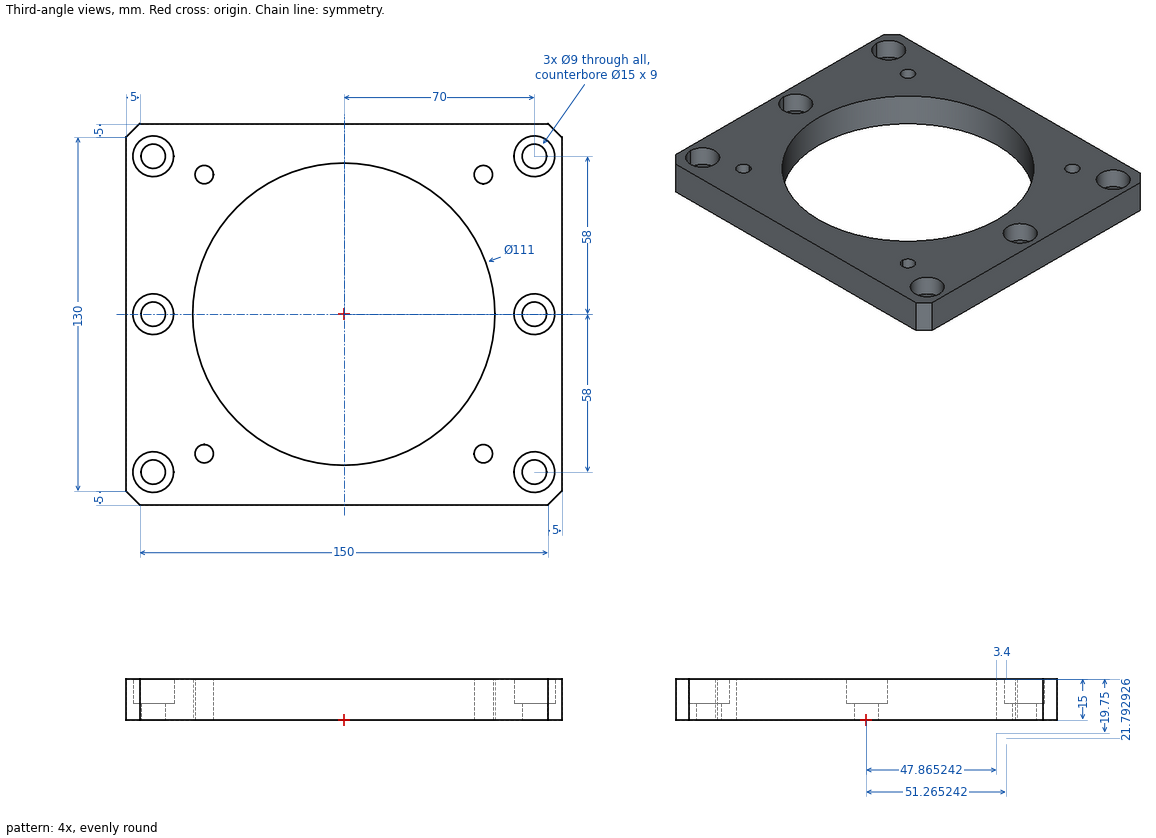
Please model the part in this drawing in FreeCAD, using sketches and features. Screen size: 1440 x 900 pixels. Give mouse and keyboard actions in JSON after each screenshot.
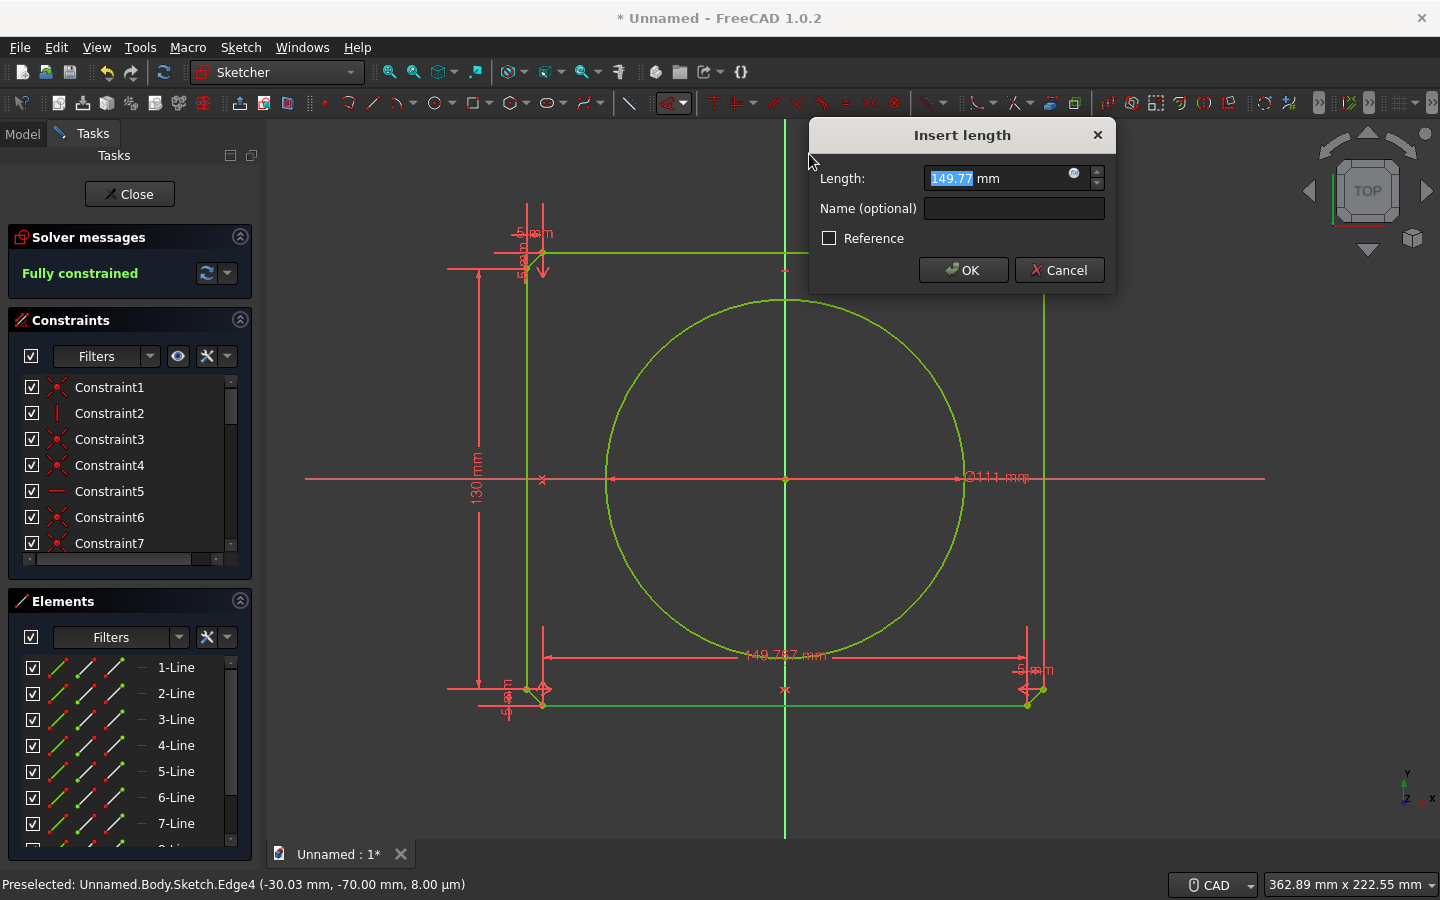
{"action": "type", "text": "150"}
{"action": "key", "text": "Return"}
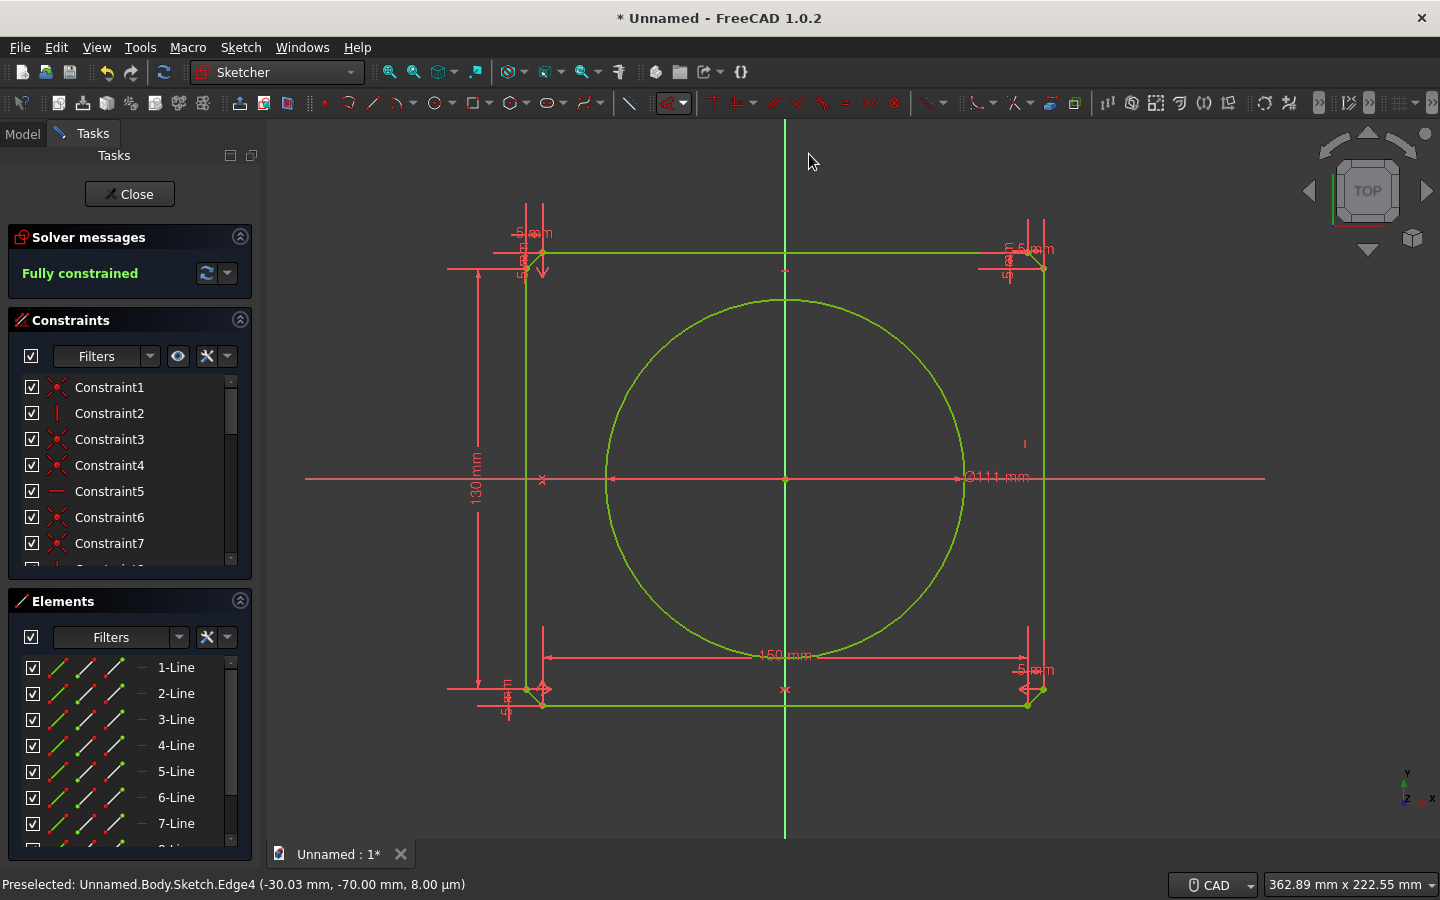
{"action": "left_click", "coordinate": [130, 194]}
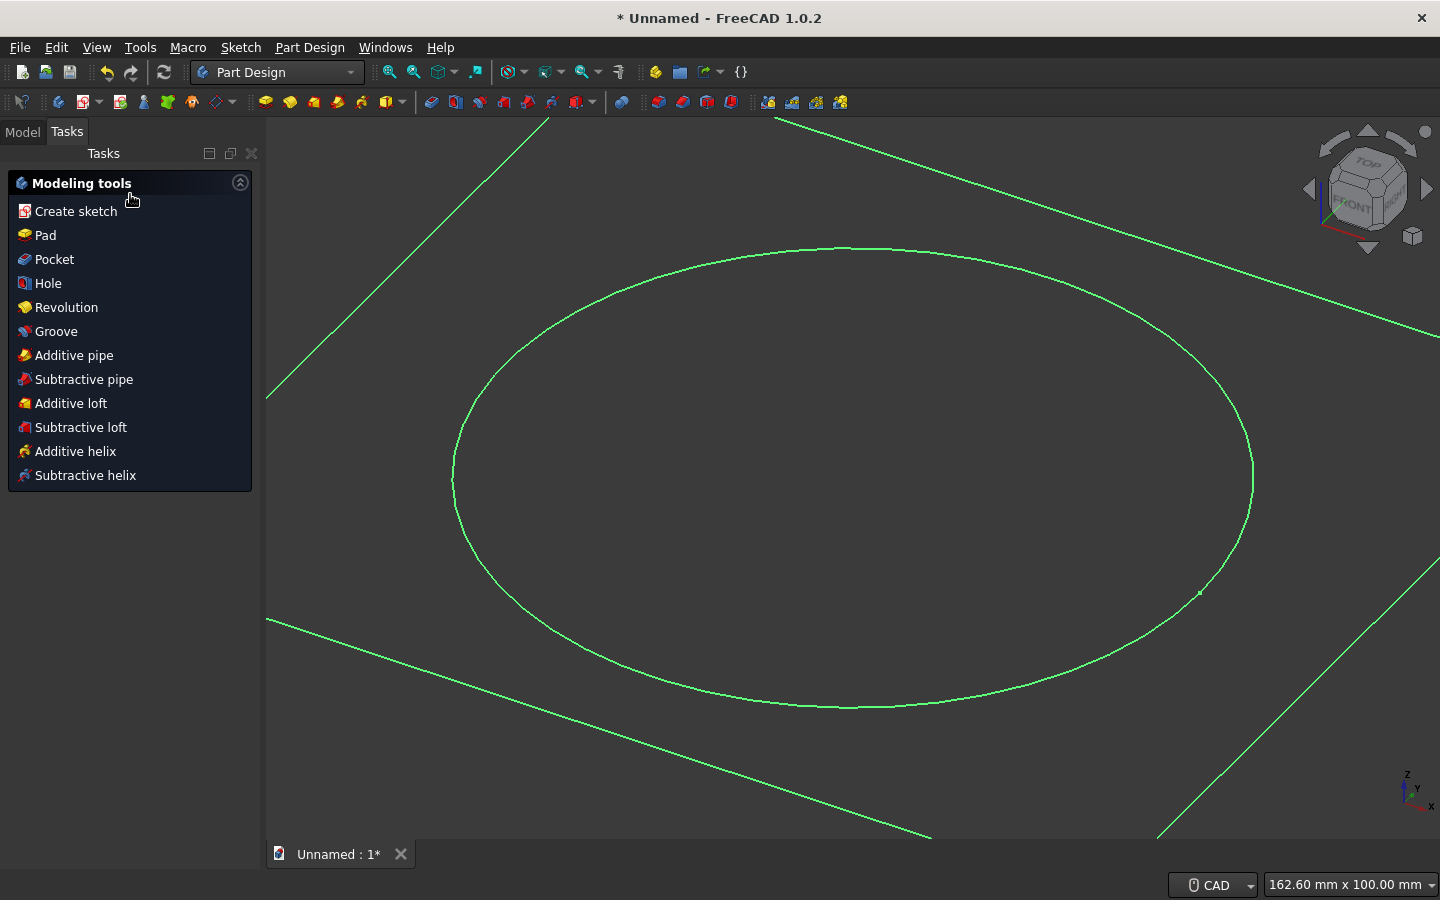
{"action": "left_click", "coordinate": [266, 102]}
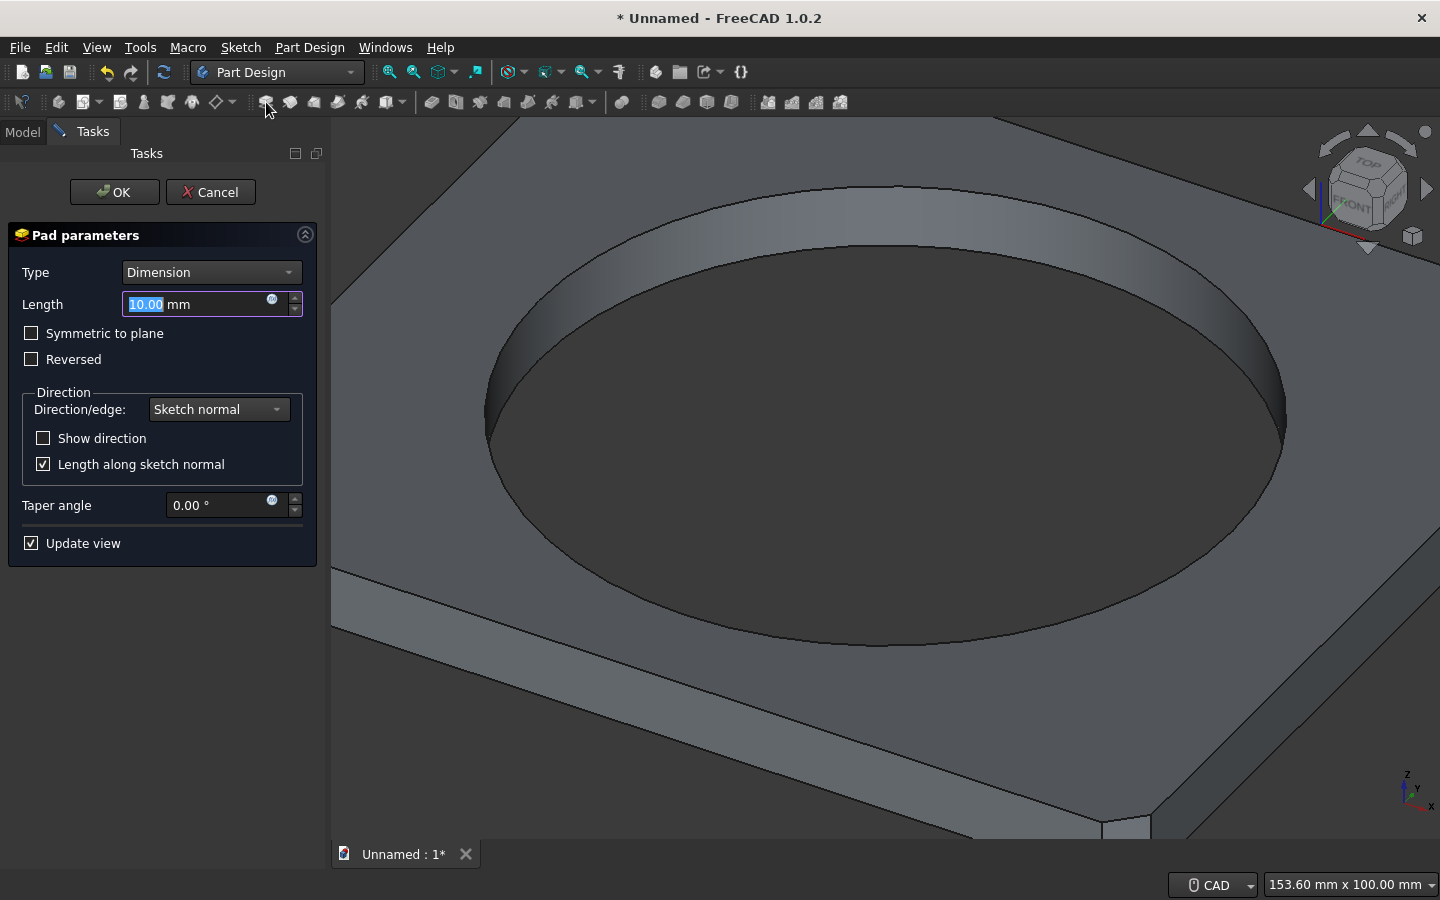
{"action": "type", "text": "15"}
{"action": "key", "text": "Tab"}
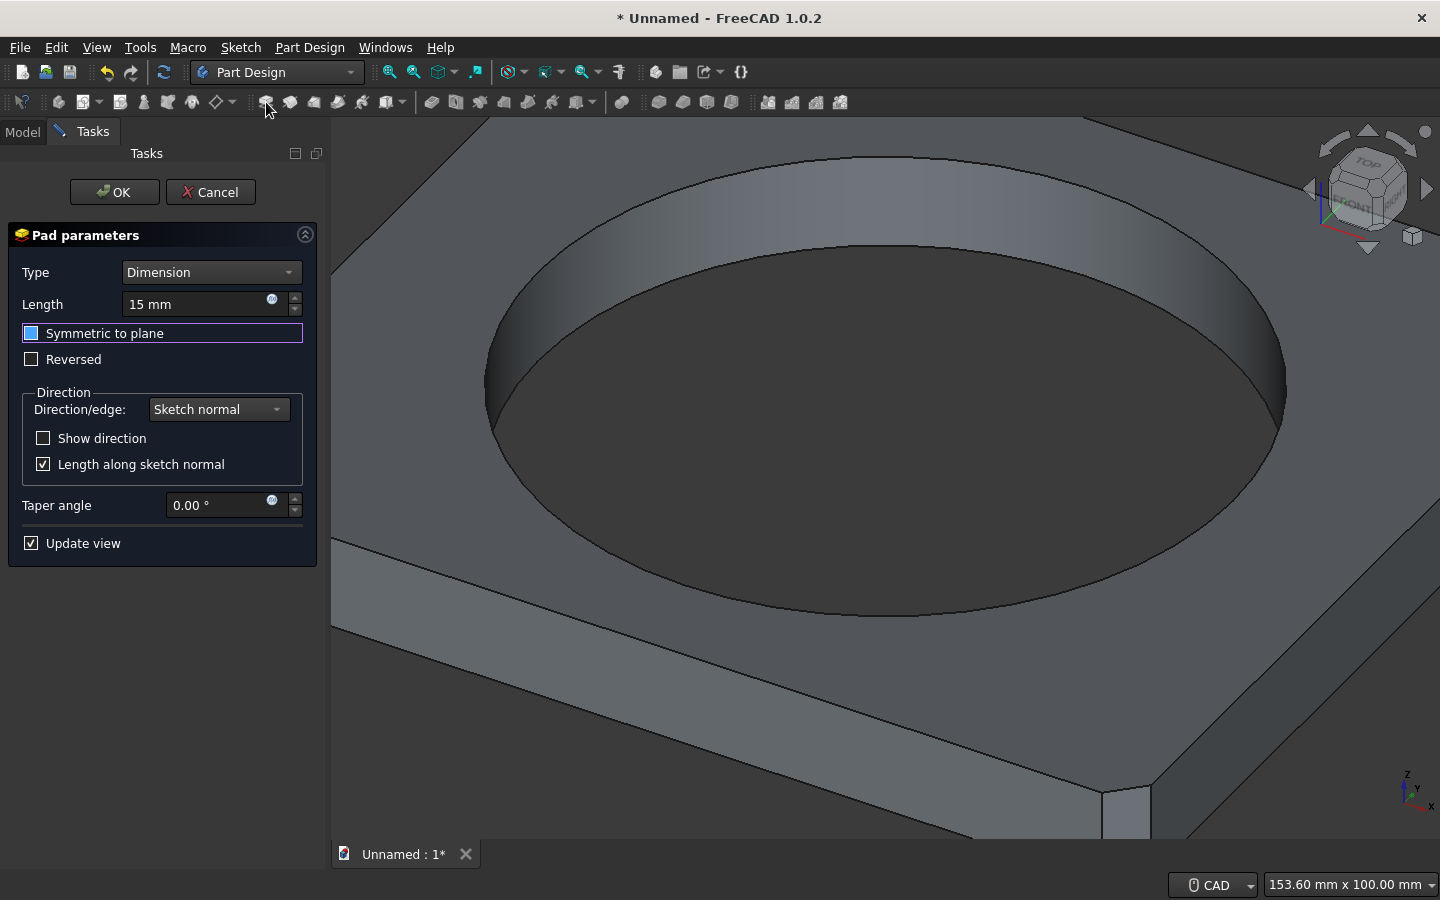
{"action": "left_click", "coordinate": [115, 192]}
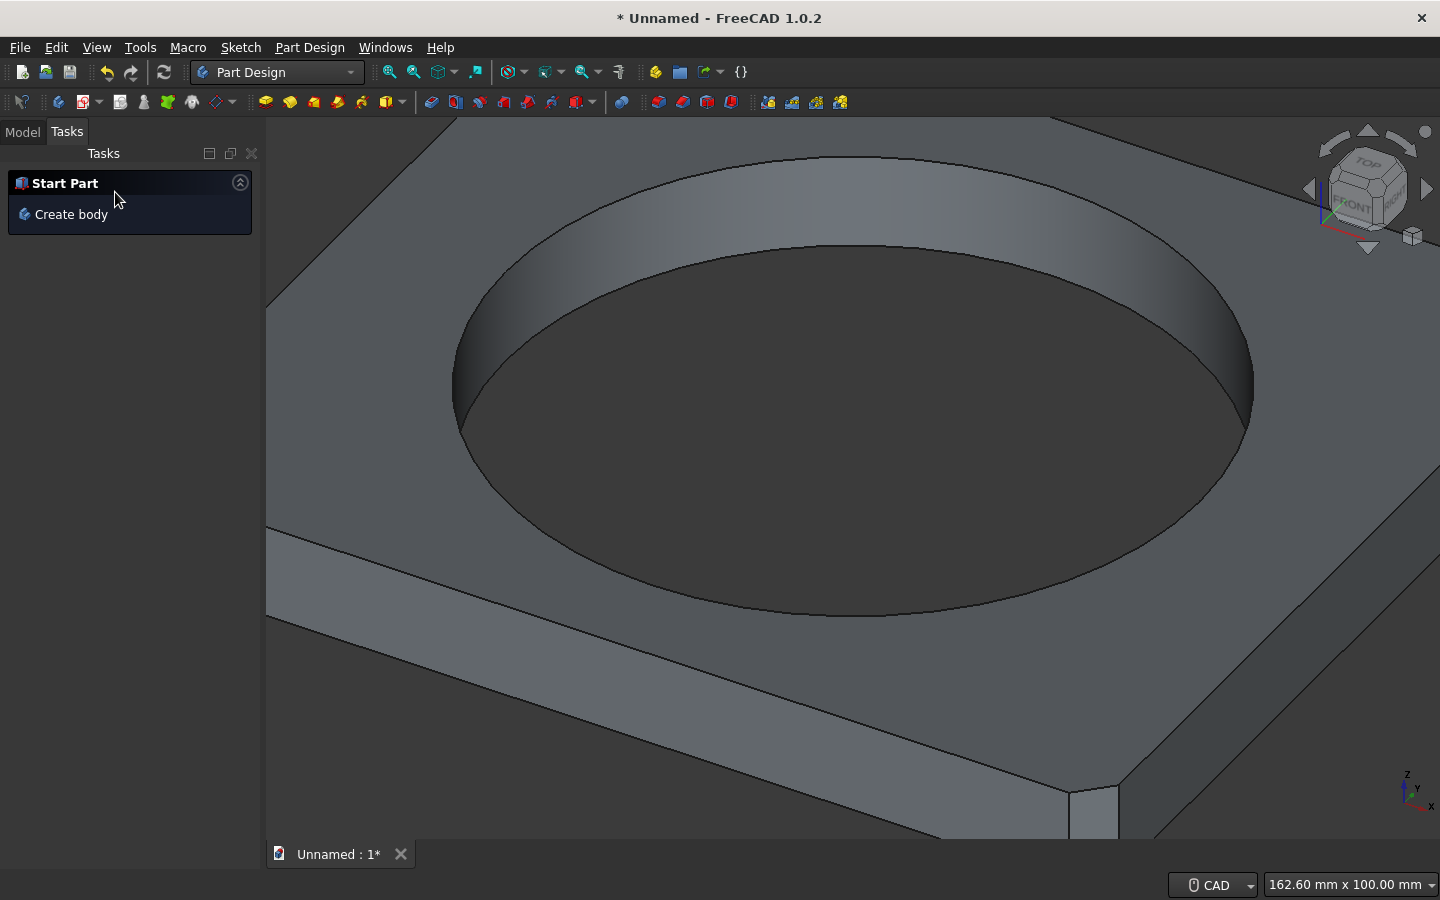
{"action": "left_click", "coordinate": [390, 72]}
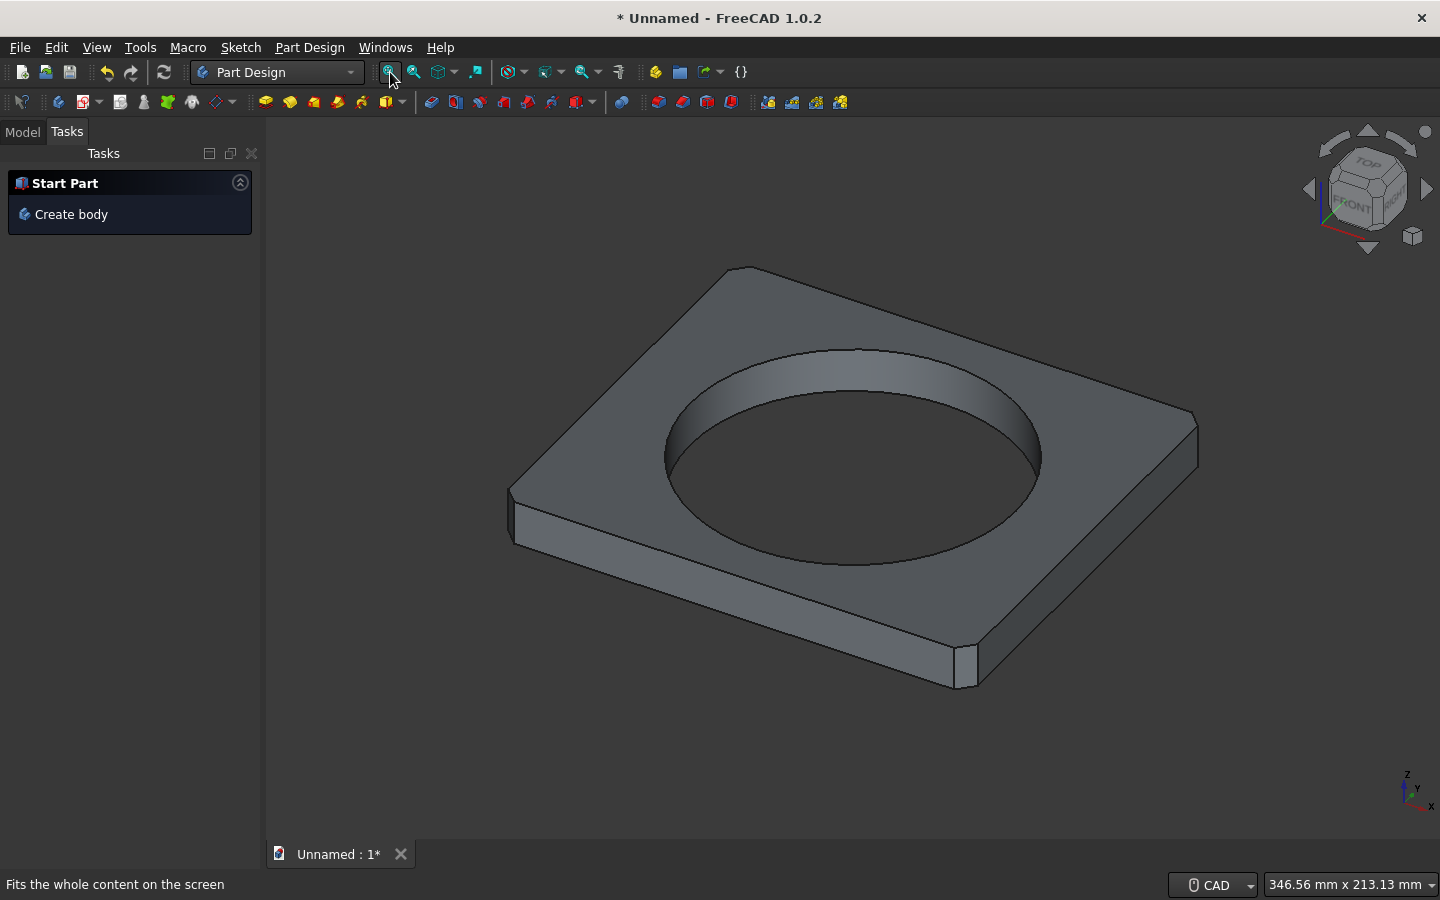
{"action": "left_click", "coordinate": [23, 131]}